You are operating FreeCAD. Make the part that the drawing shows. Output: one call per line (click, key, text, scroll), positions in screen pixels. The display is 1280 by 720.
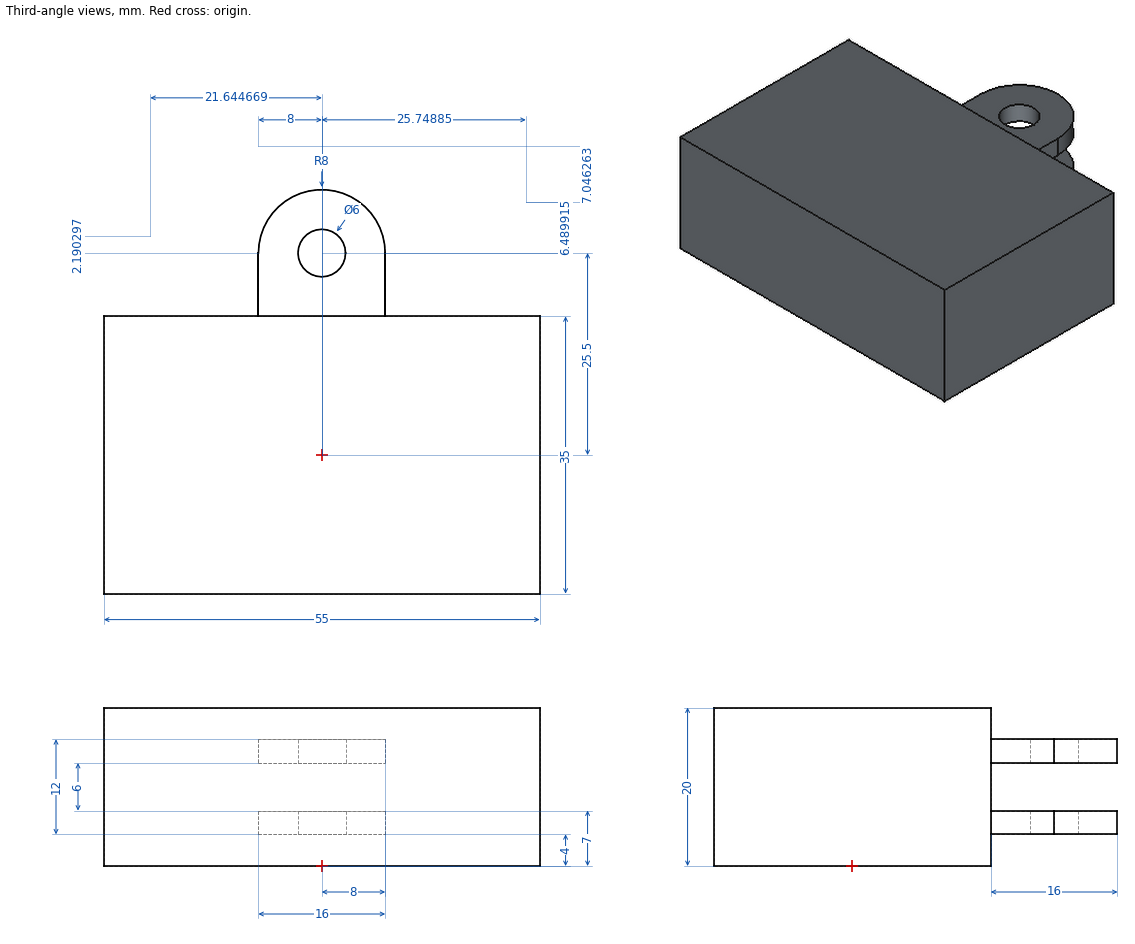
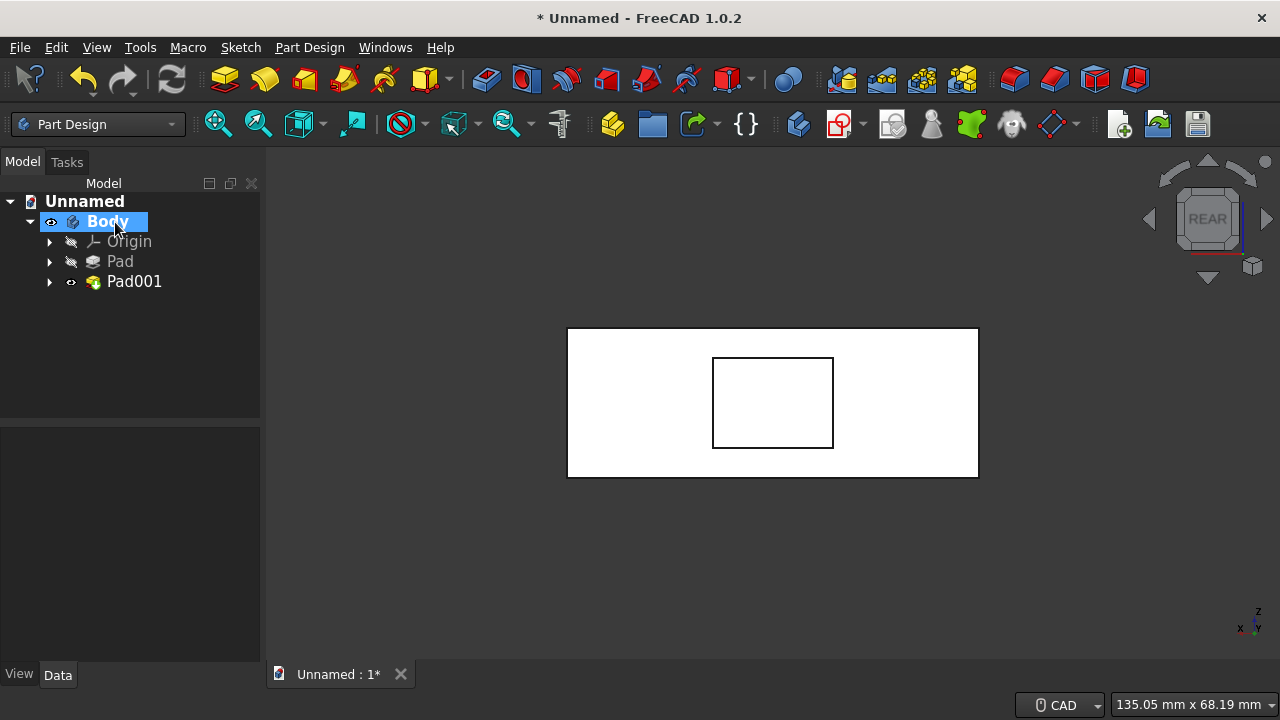
click(220, 124)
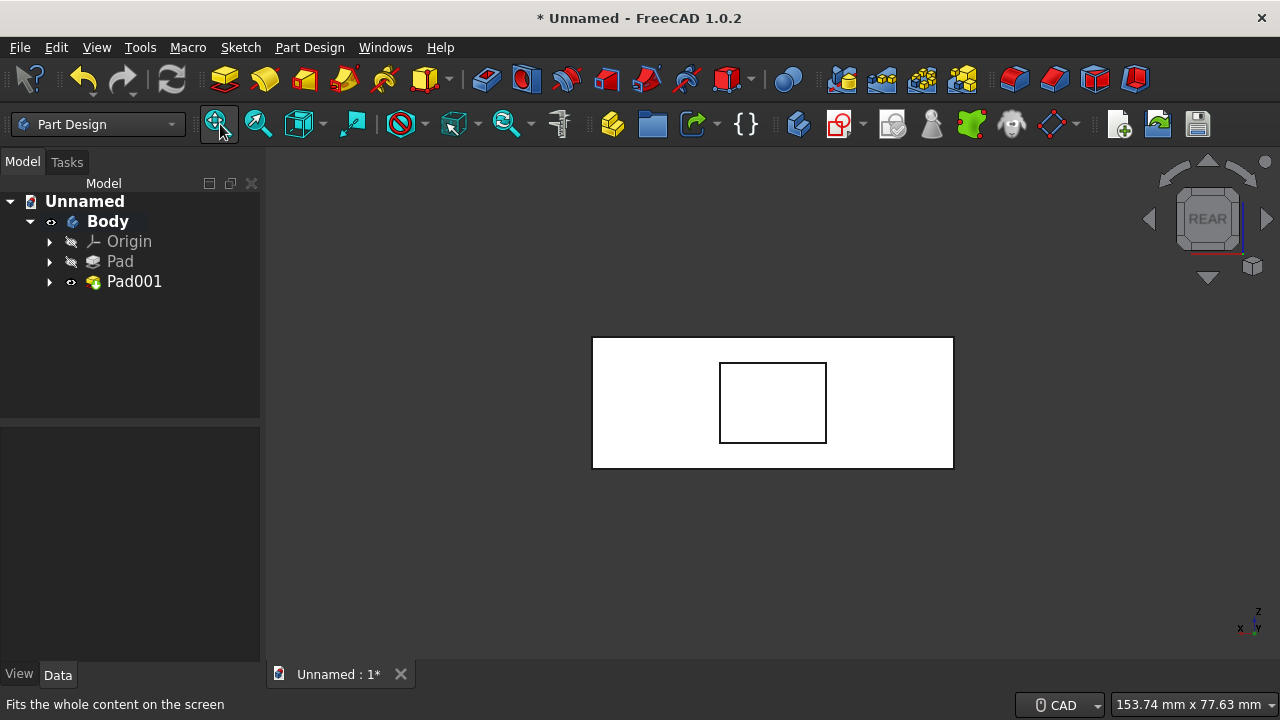
click(773, 402)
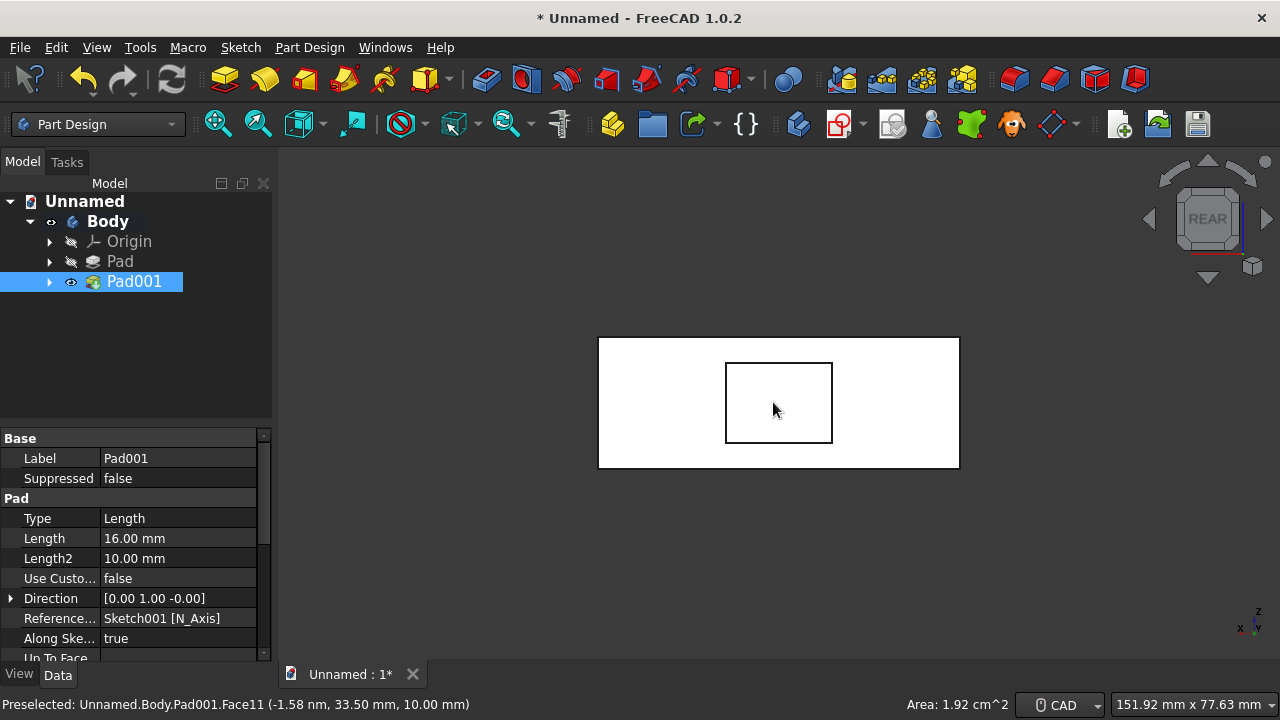
click(840, 124)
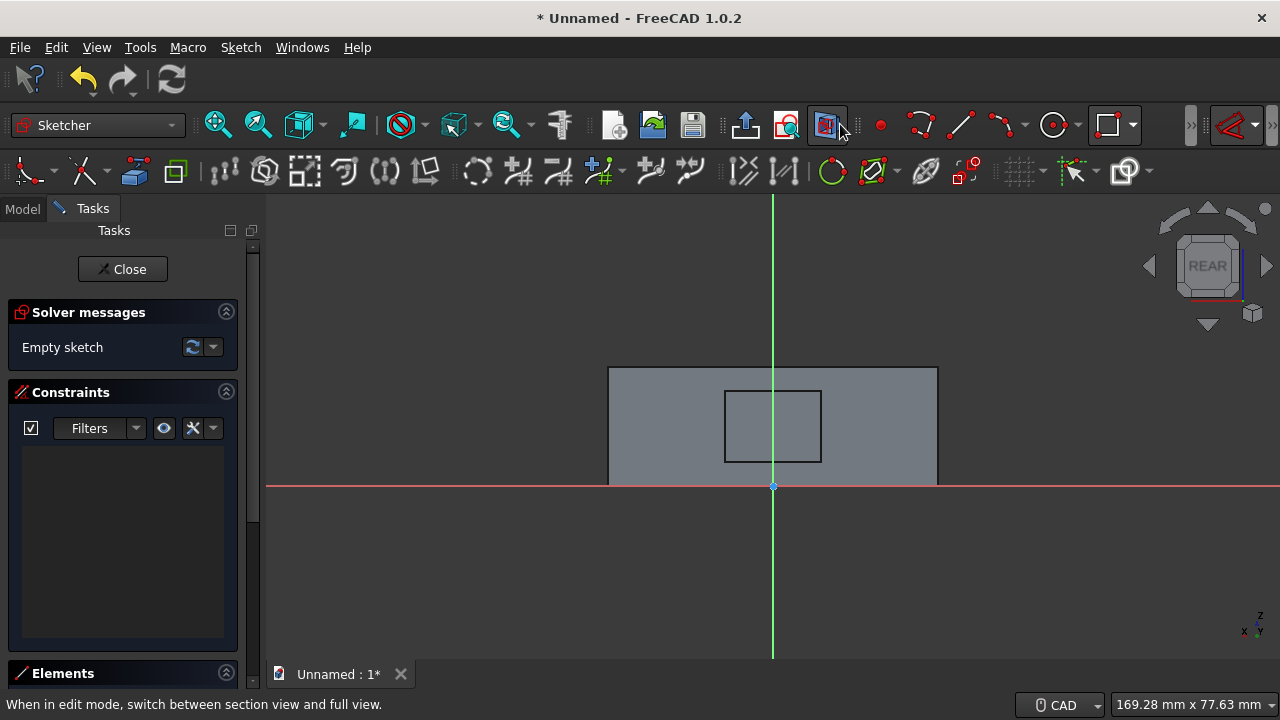
scroll(795, 454, up, 7)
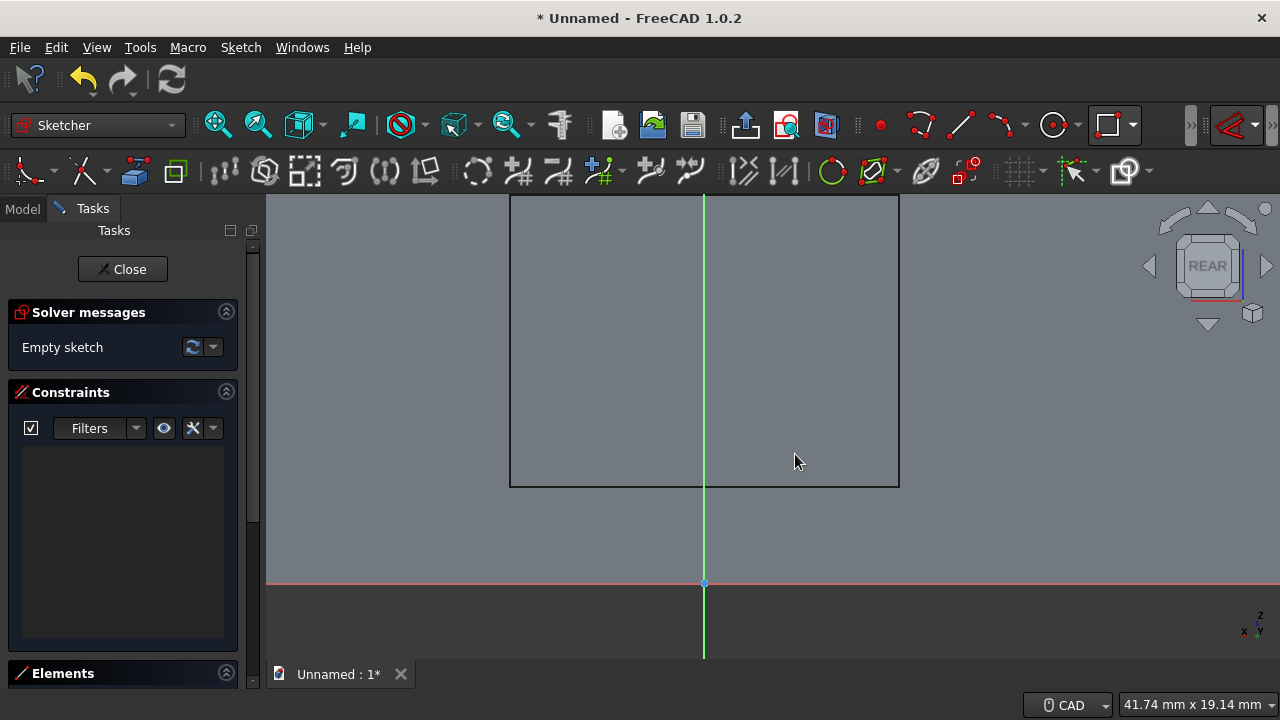
key(g)
key(r)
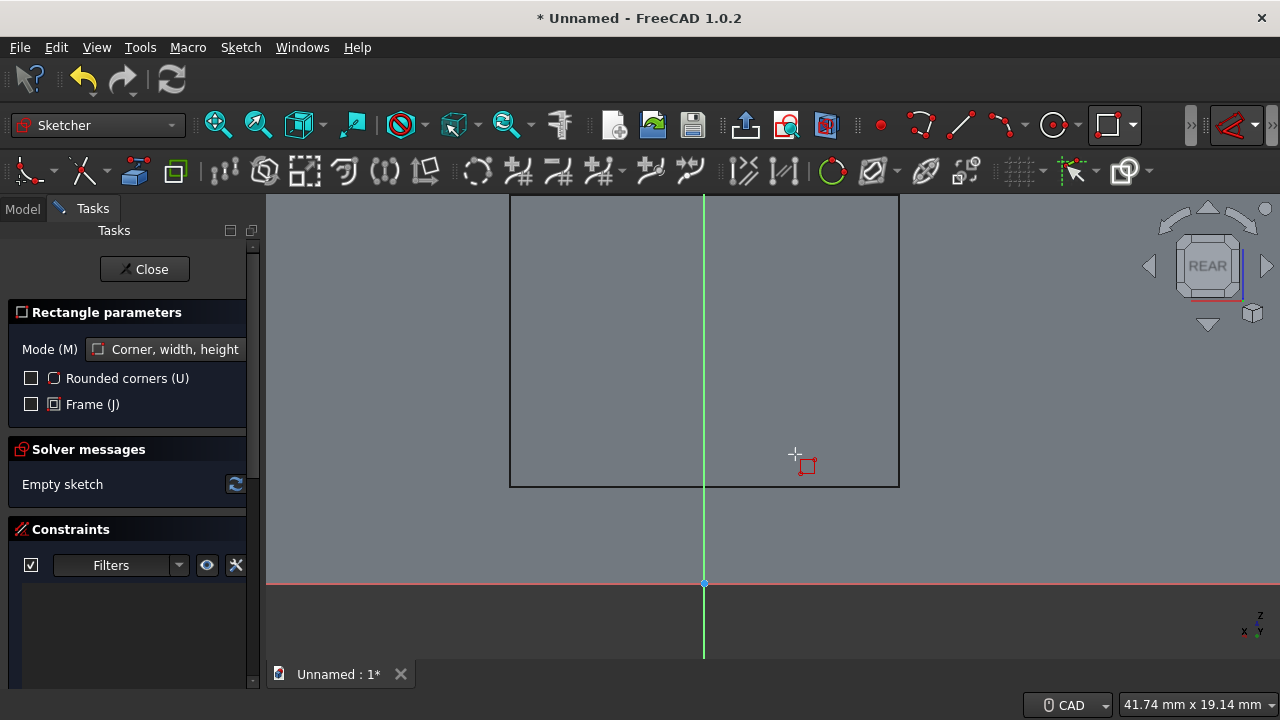
click(510, 268)
move(899, 414)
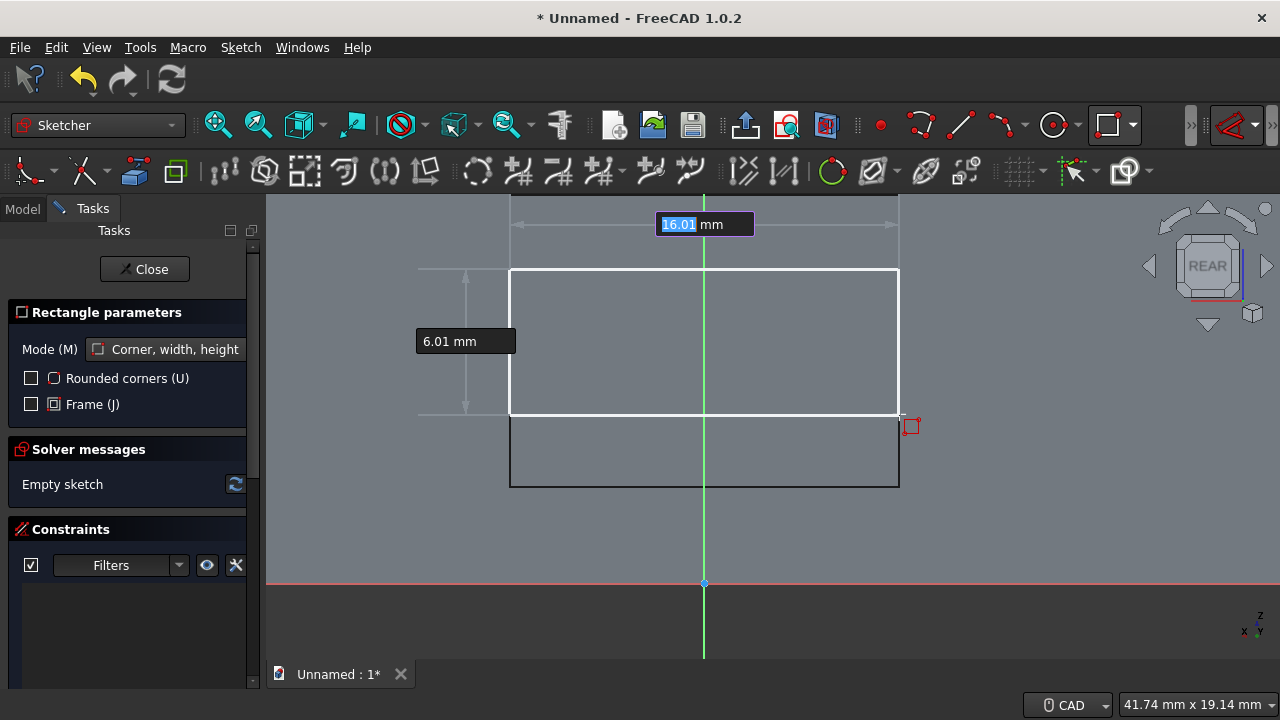
text(16)
key(Tab)
text(6)
key(Return)
key(Escape)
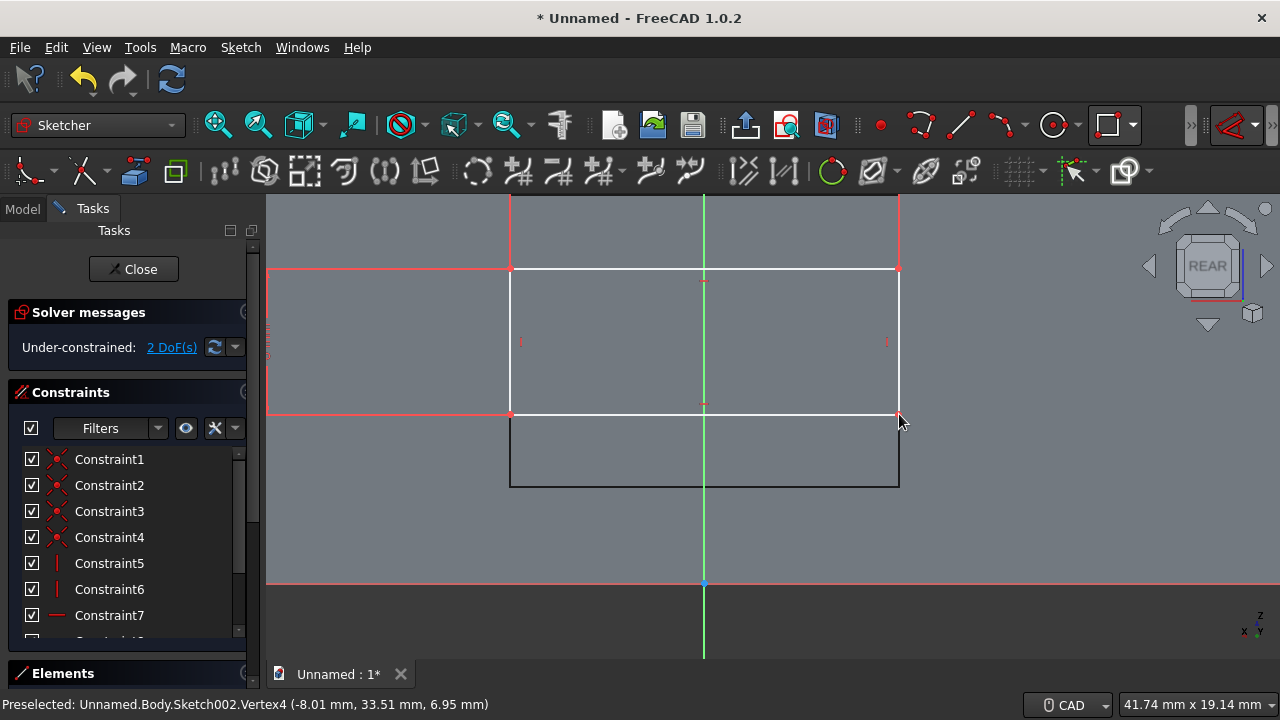
click(510, 269)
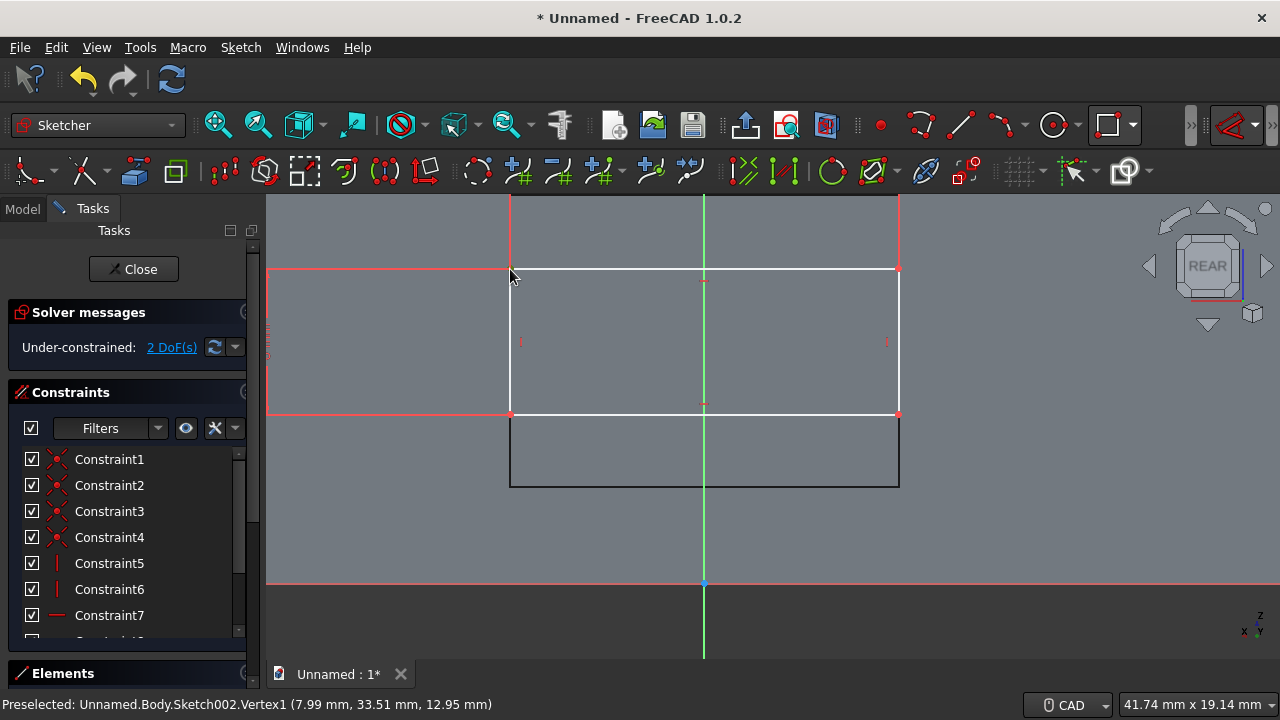
click(1258, 126)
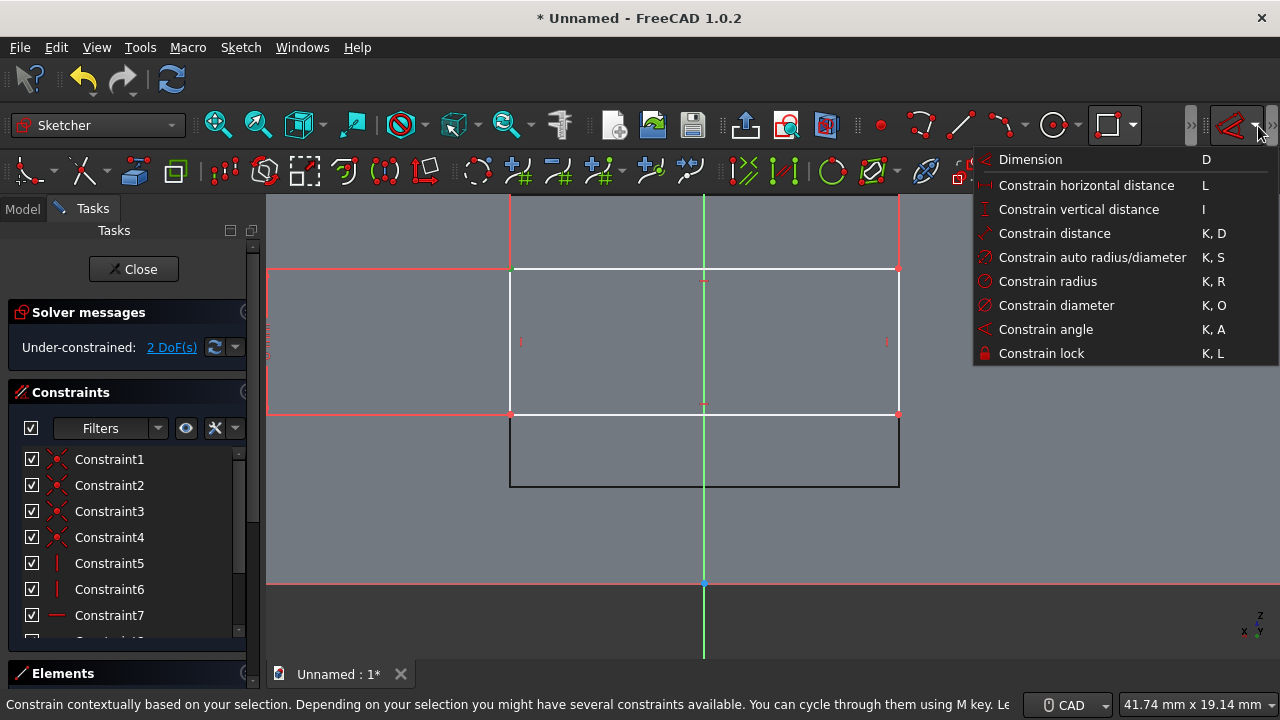
click(1126, 185)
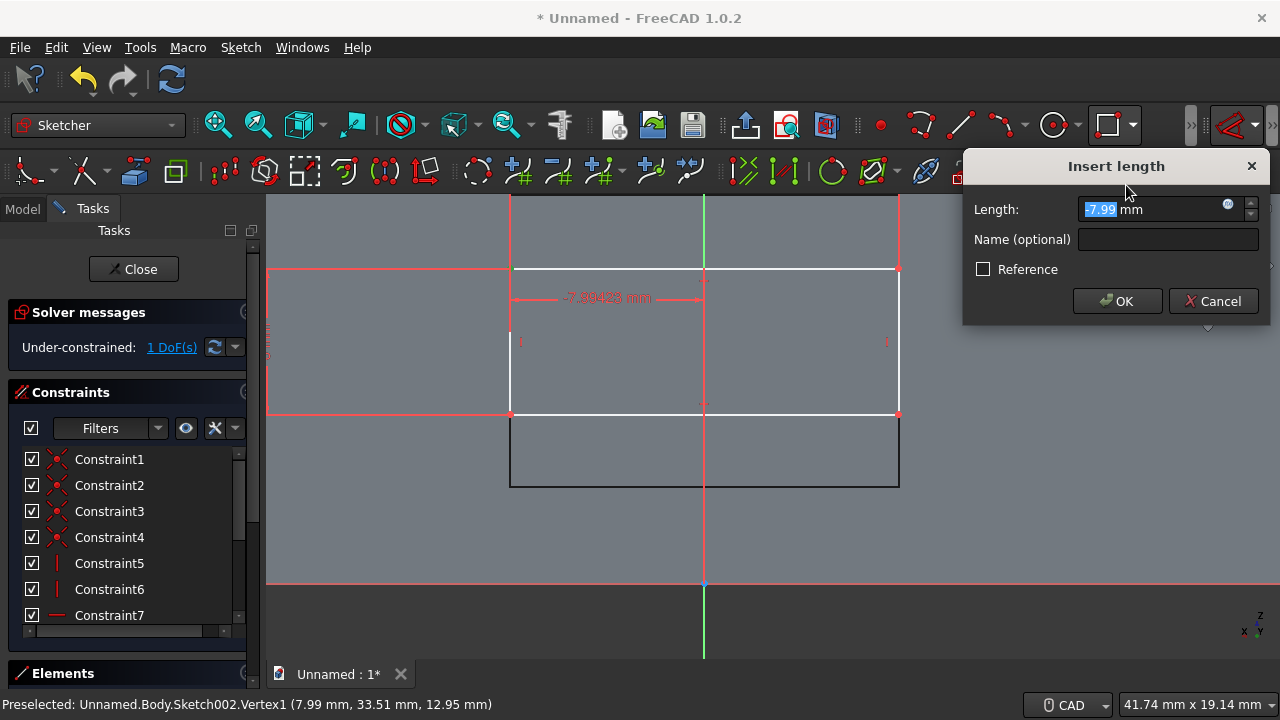
text(-8)
key(Return)